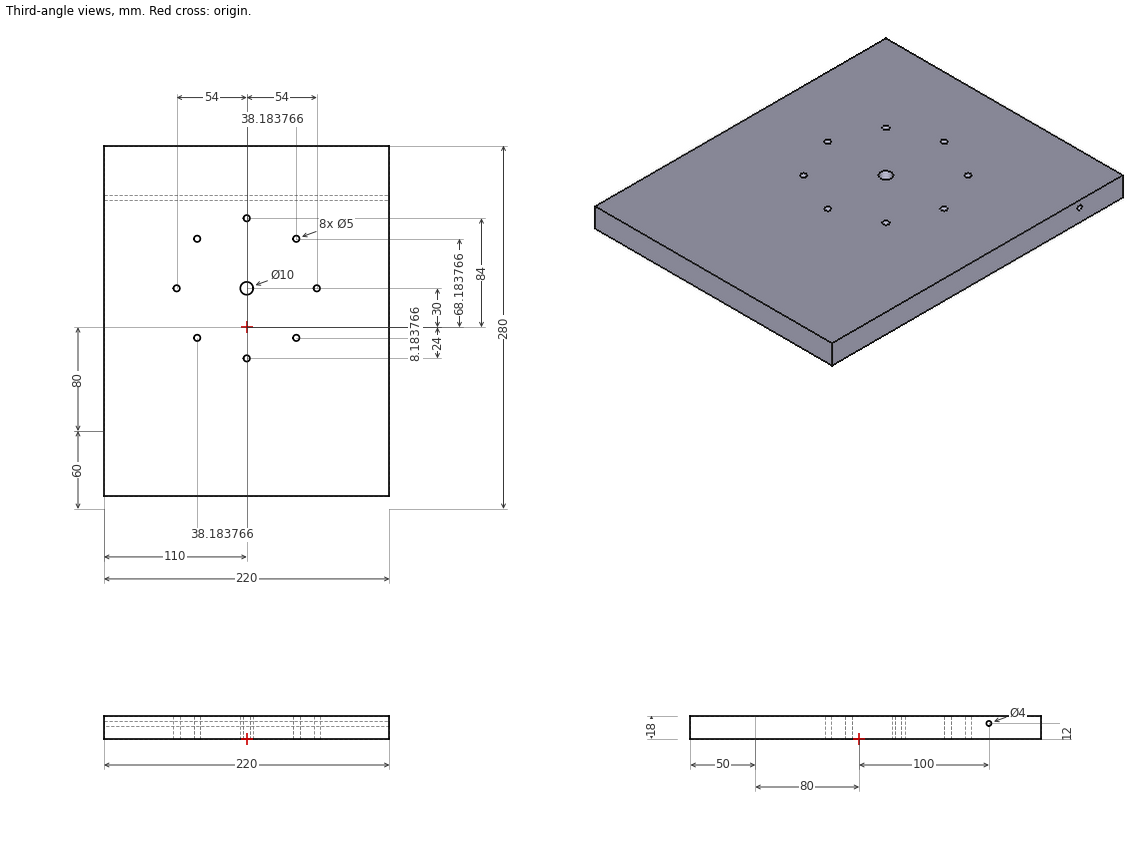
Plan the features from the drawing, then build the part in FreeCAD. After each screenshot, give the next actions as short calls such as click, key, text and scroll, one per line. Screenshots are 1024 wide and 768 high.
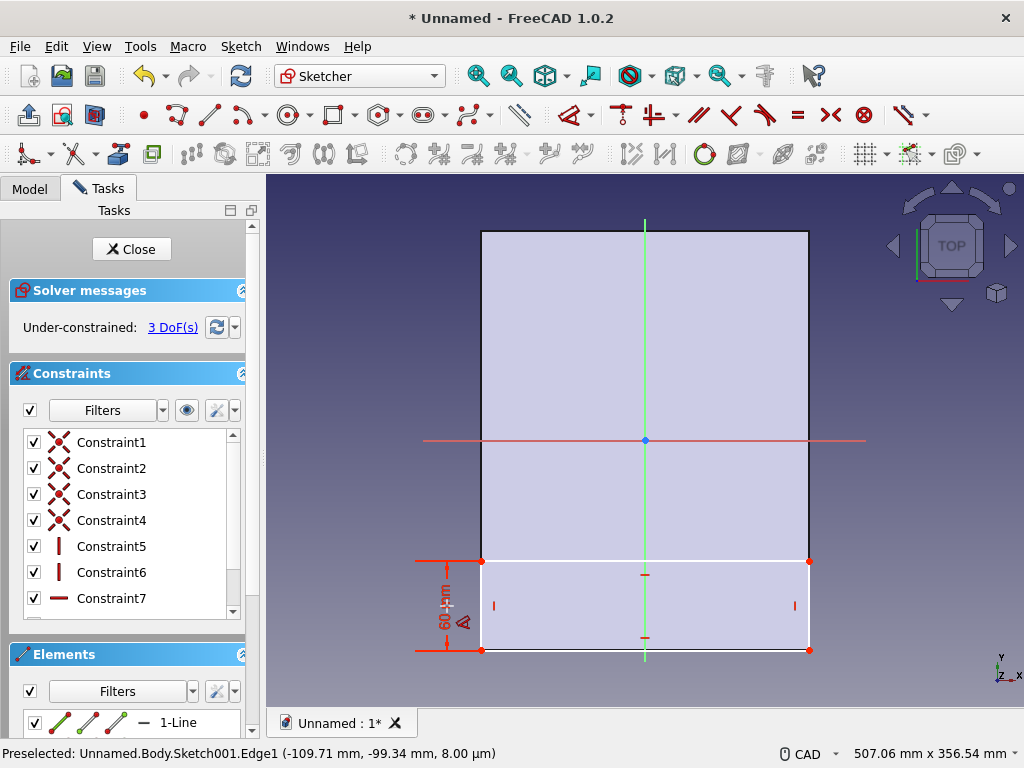
click(579, 651)
click(570, 617)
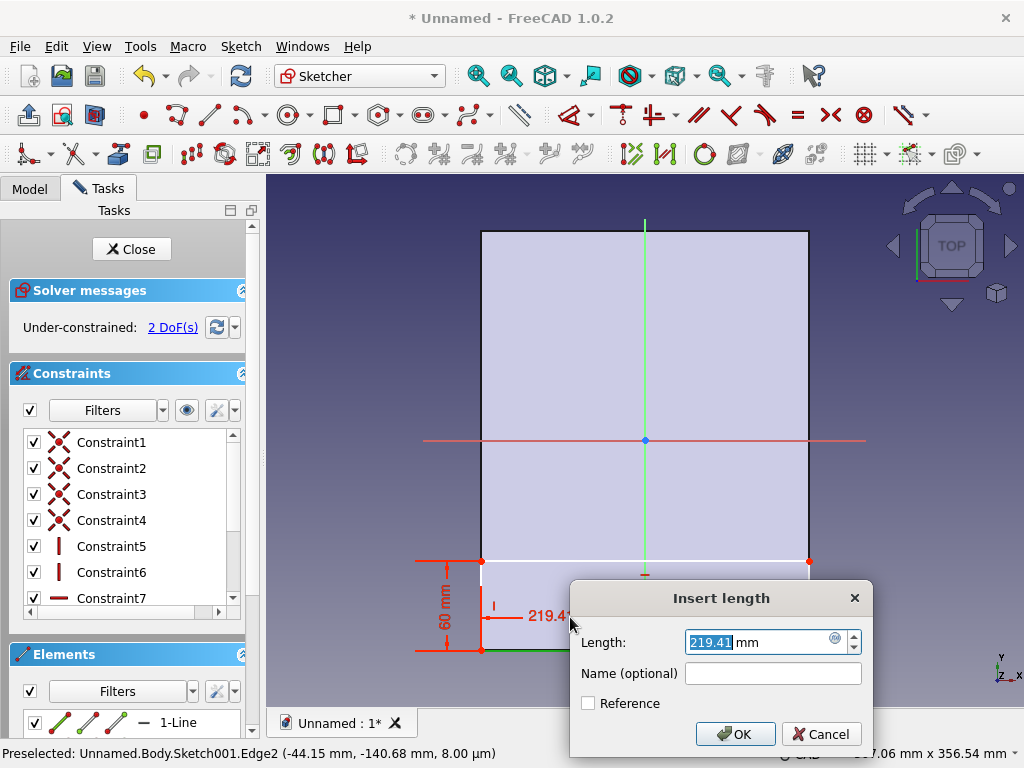
text(220)
key(Return)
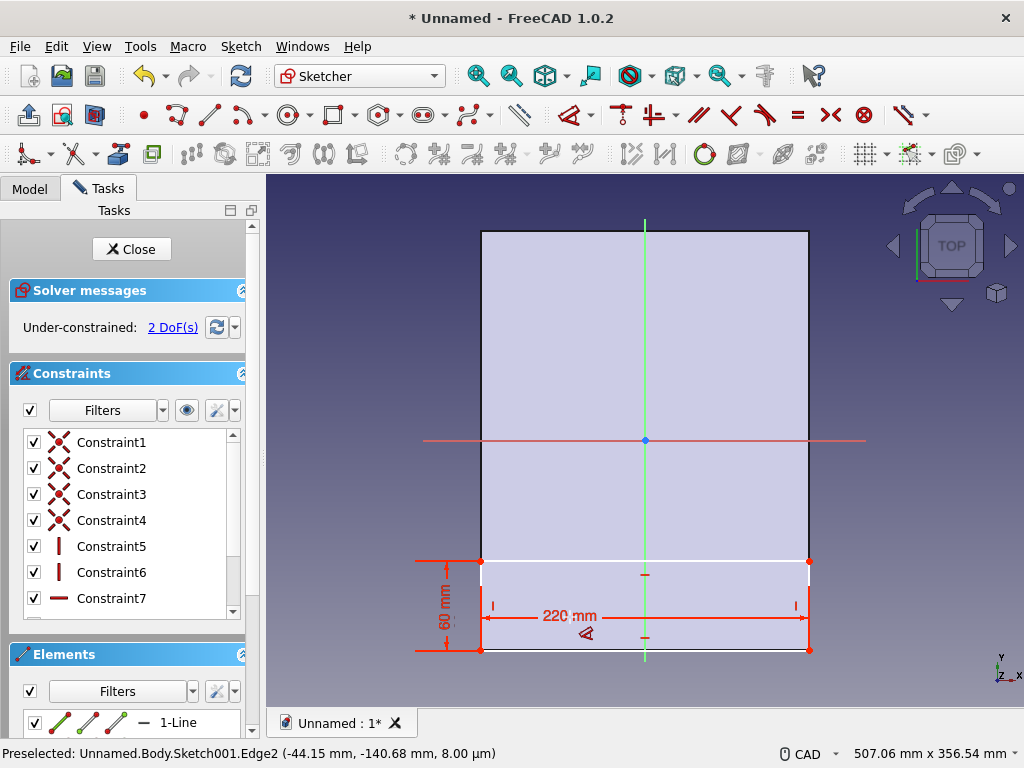
click(481, 561)
click(447, 501)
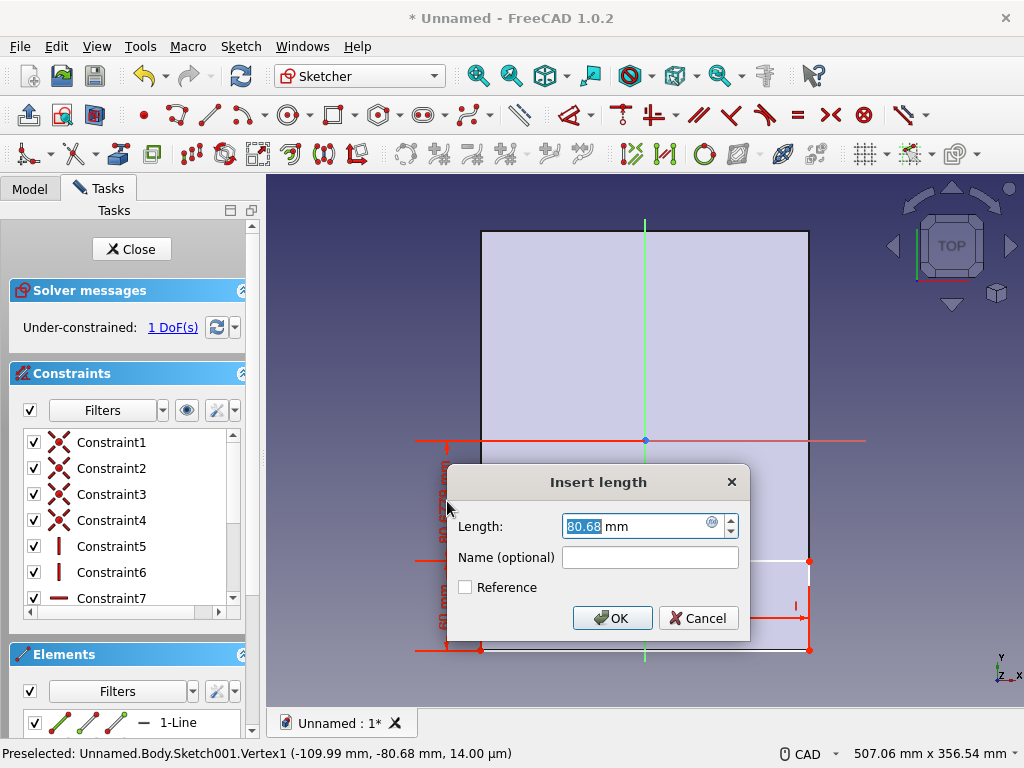
text(80)
key(Return)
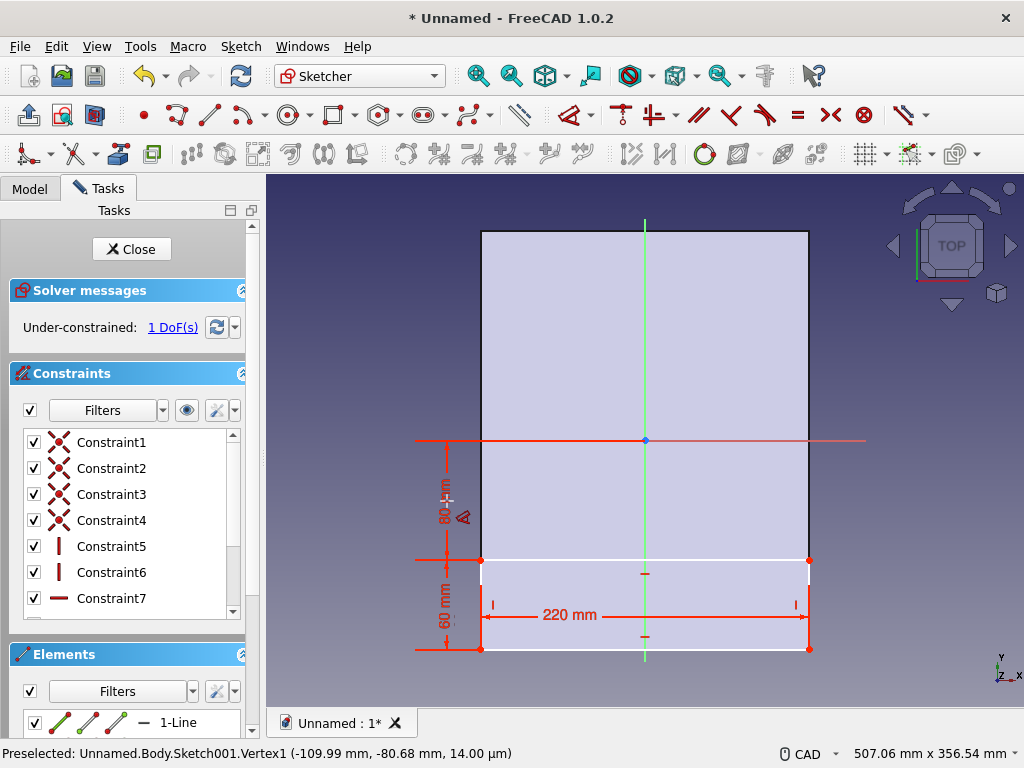
click(481, 560)
click(563, 406)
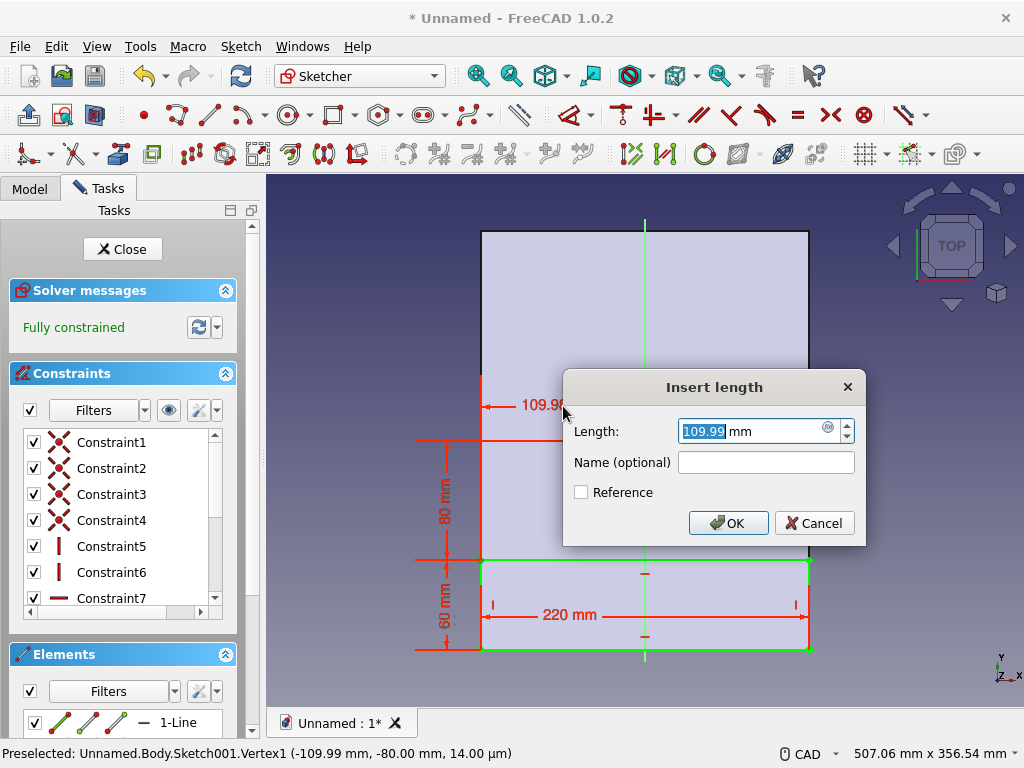
text(110)
key(Return)
key(Escape)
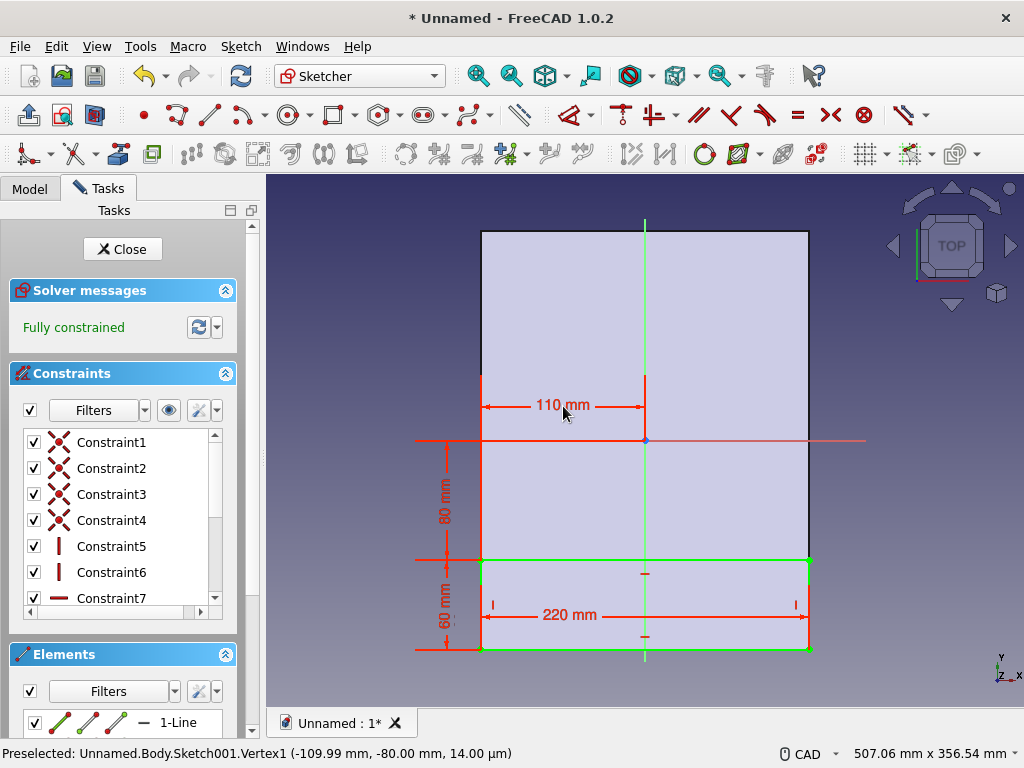
click(123, 249)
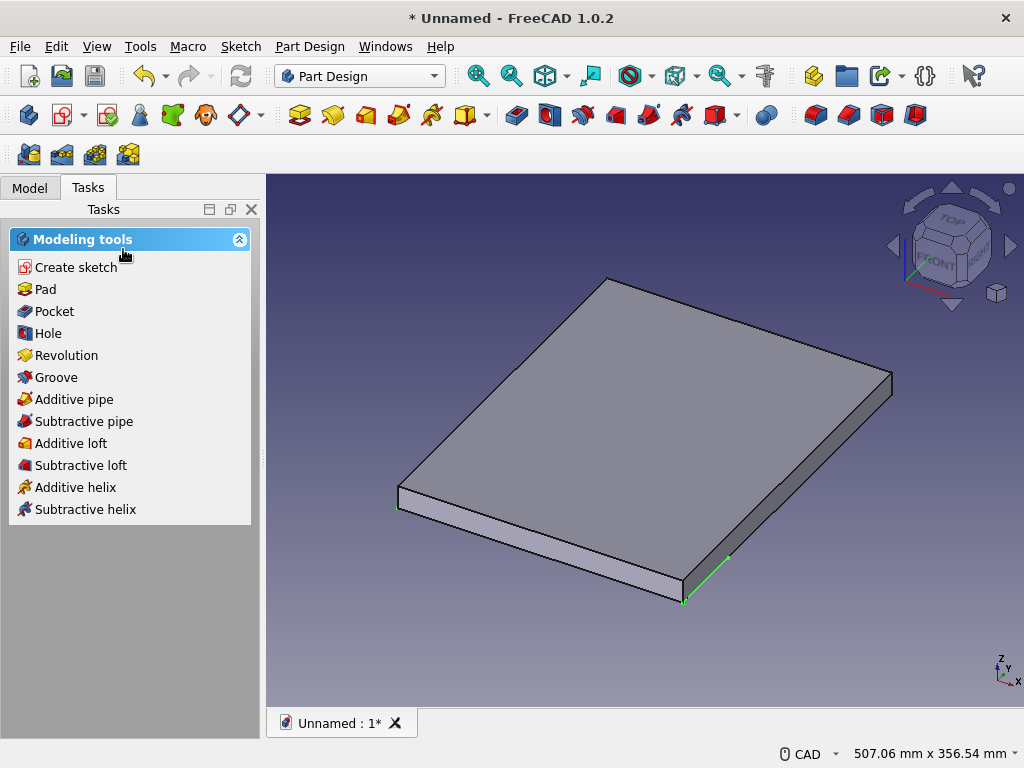
click(517, 116)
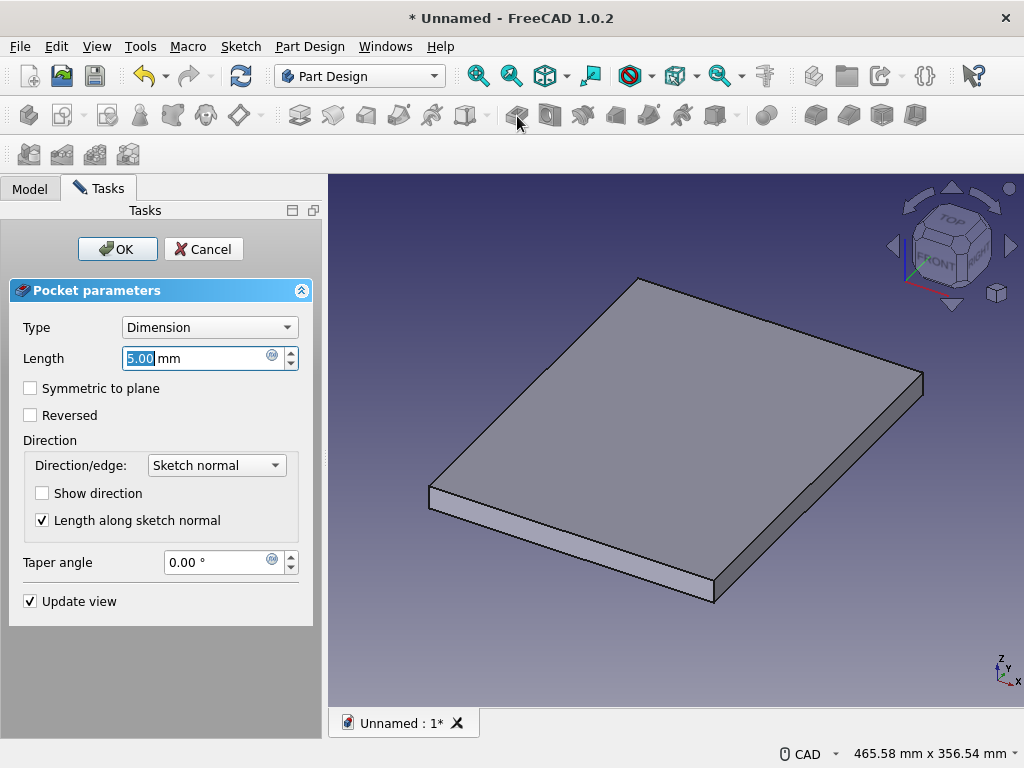
click(210, 328)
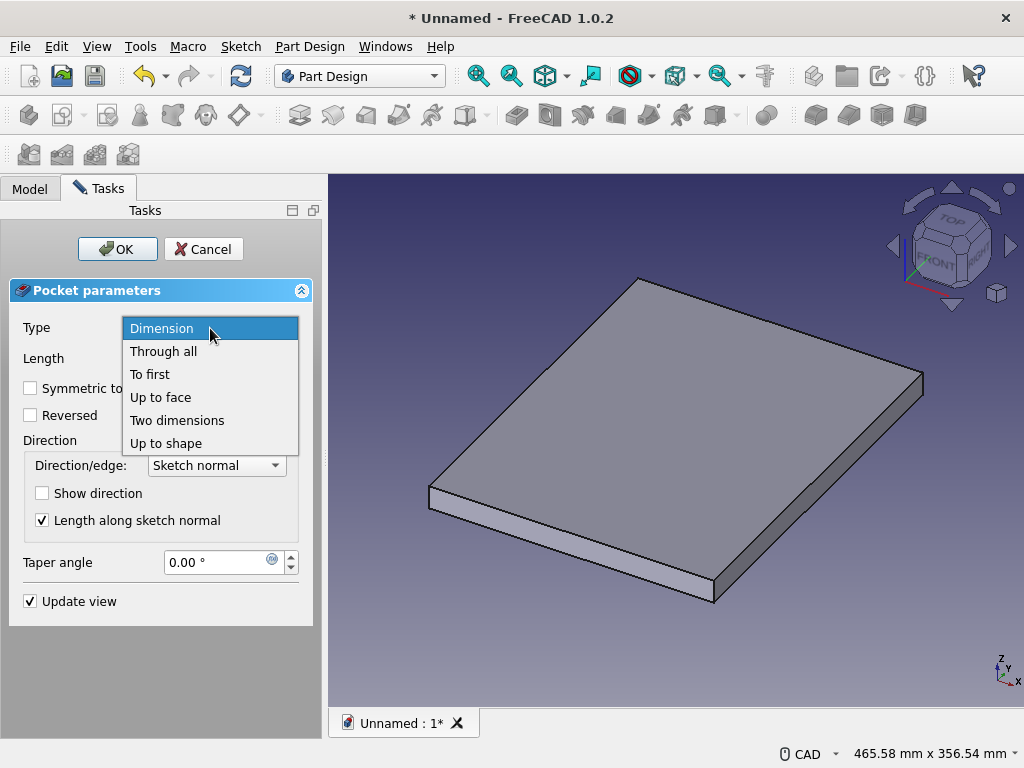
click(208, 352)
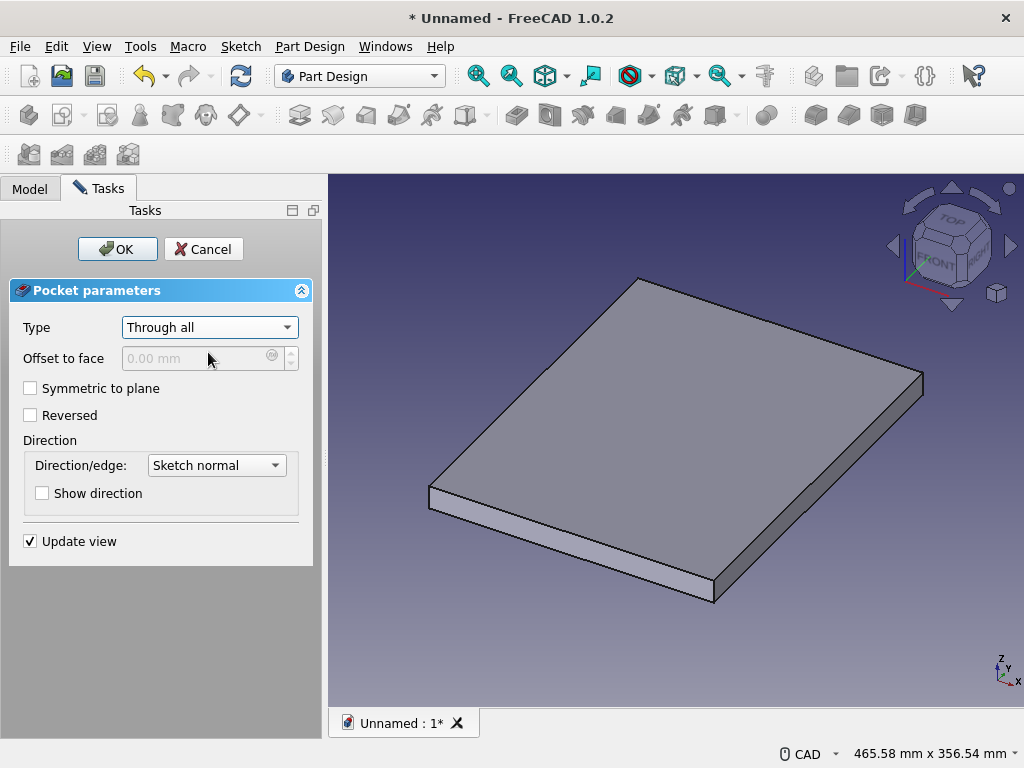
click(31, 415)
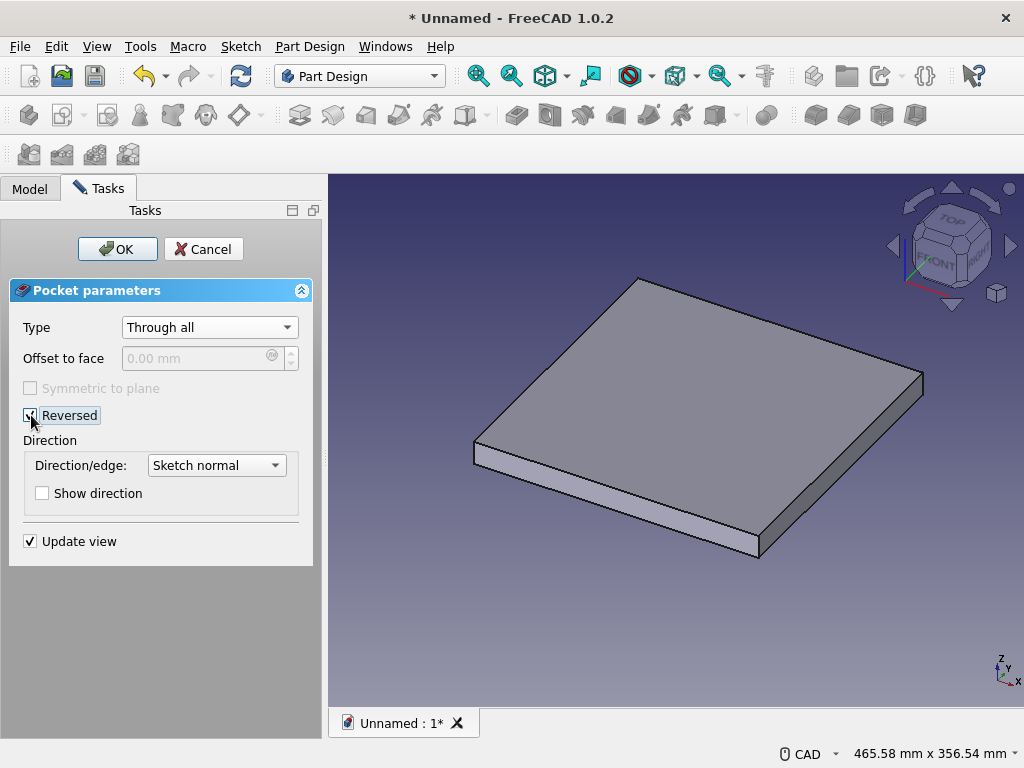
click(118, 249)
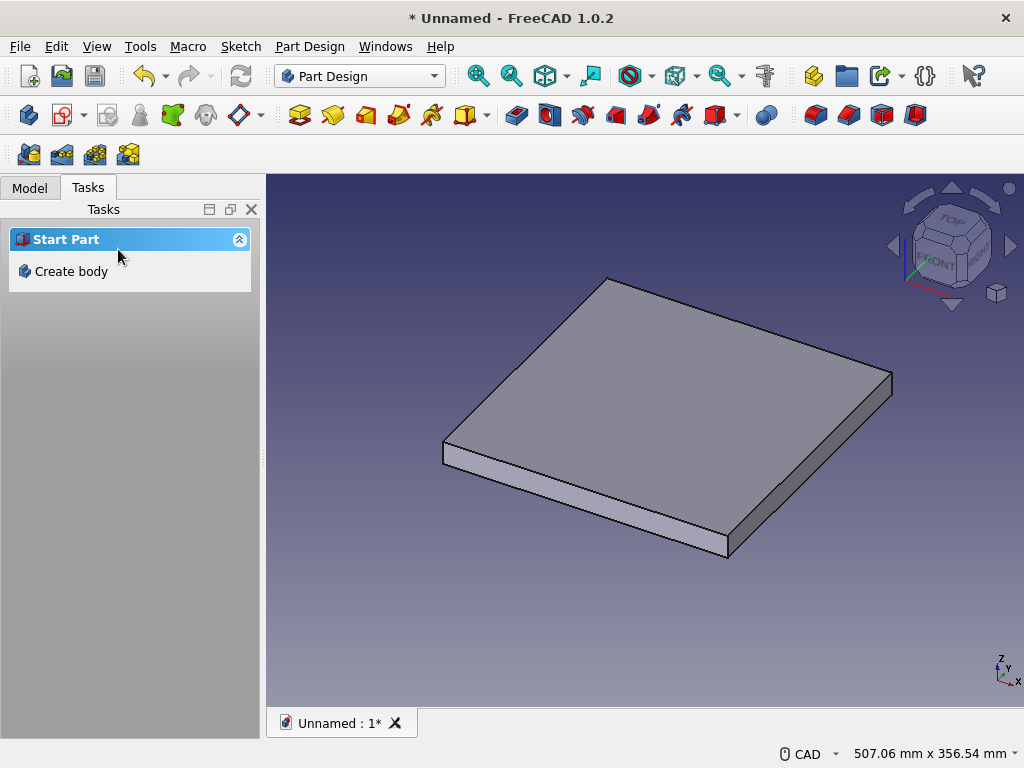
key(5)